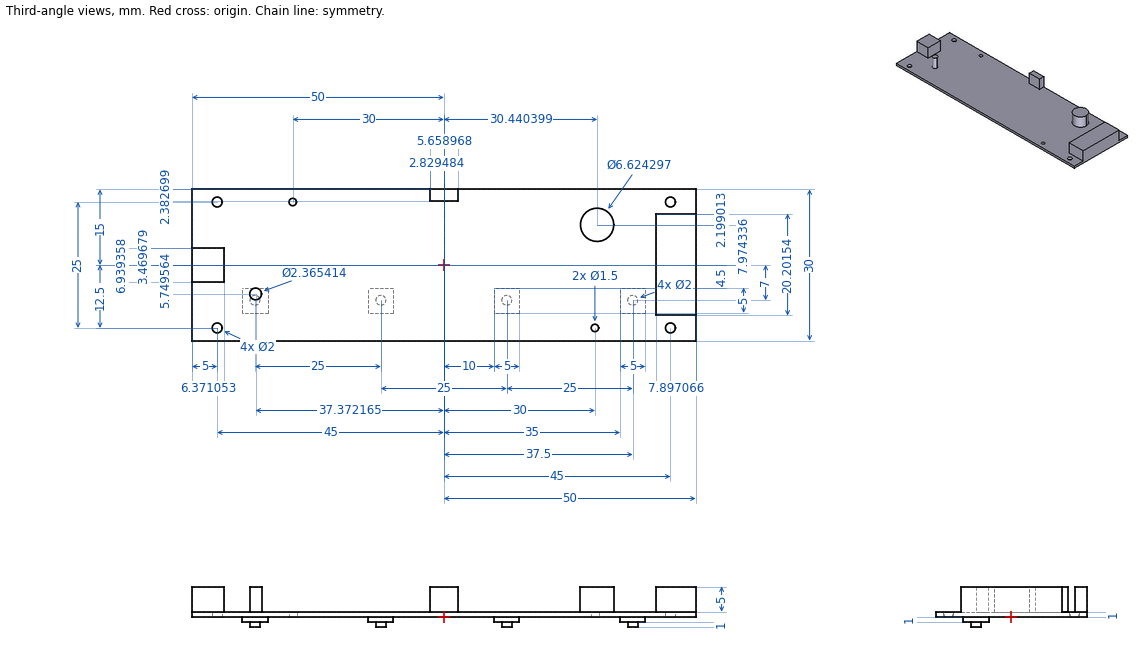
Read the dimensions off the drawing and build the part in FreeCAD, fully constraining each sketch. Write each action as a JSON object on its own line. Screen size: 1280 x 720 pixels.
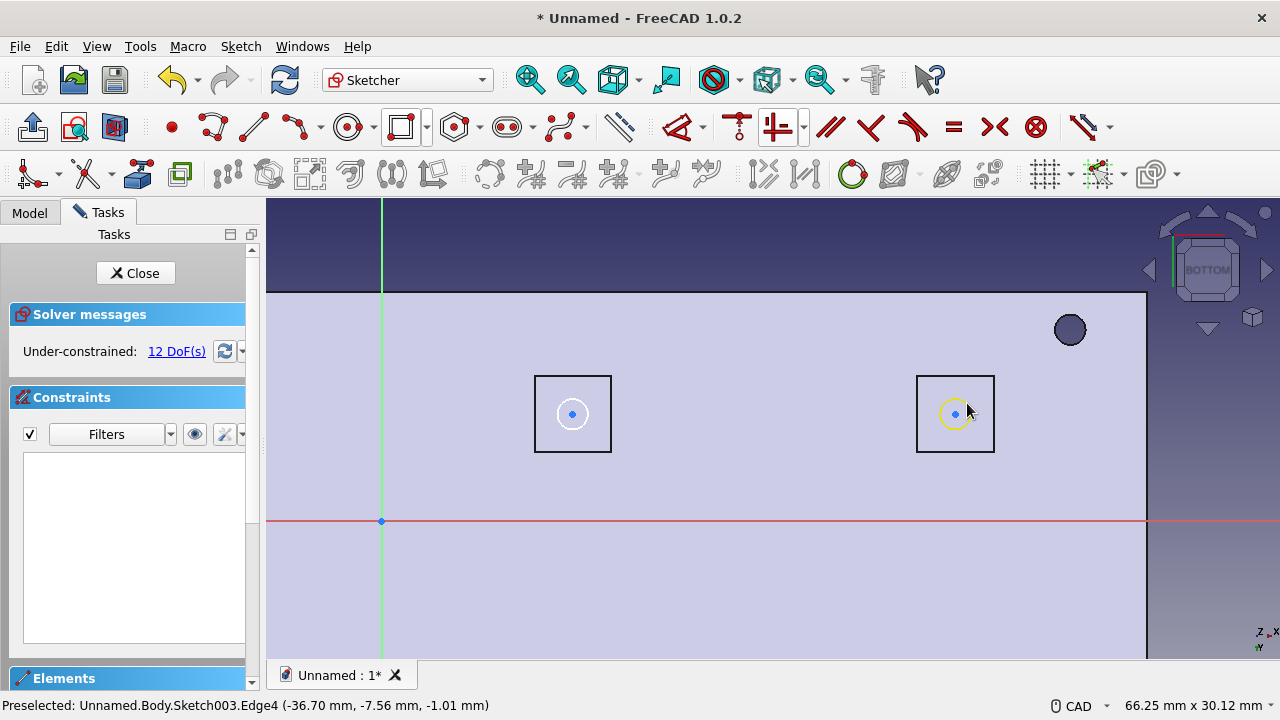
{"action": "left_click", "coordinate": [966, 404]}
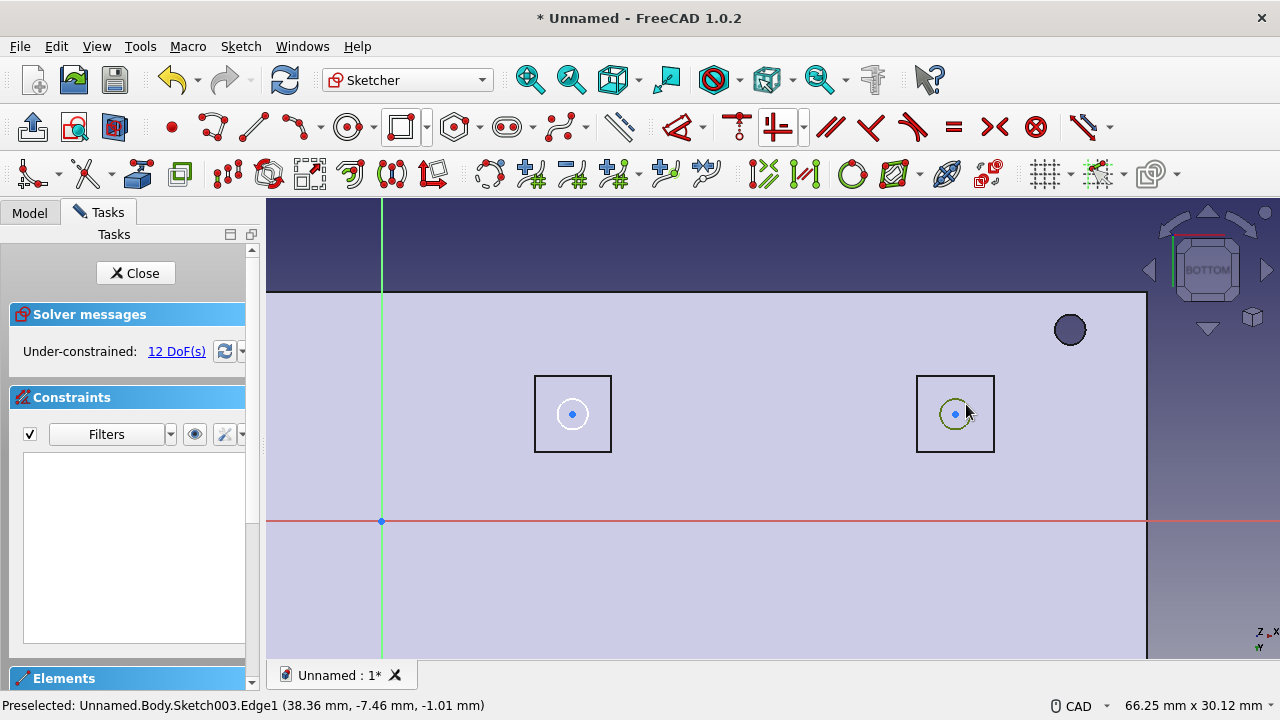
{"action": "left_click", "coordinate": [583, 404]}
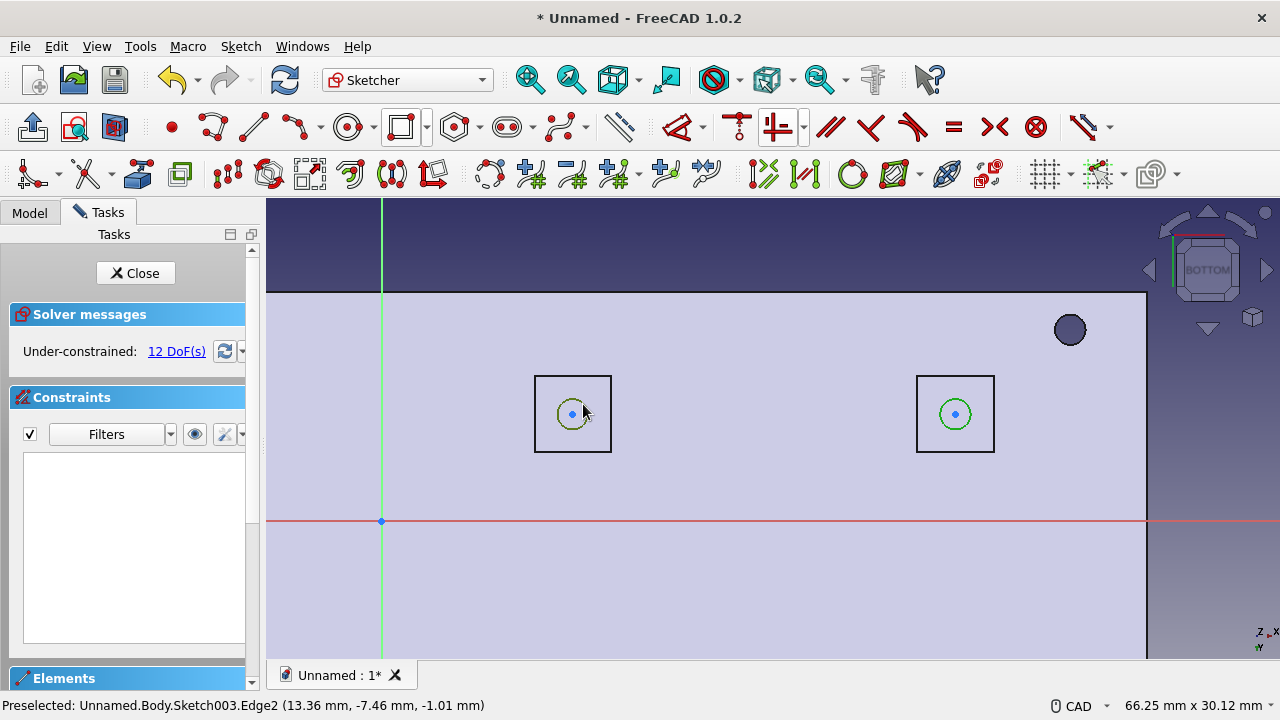
{"action": "scroll", "coordinate": [968, 403], "scroll_direction": "down", "scroll_amount": 4}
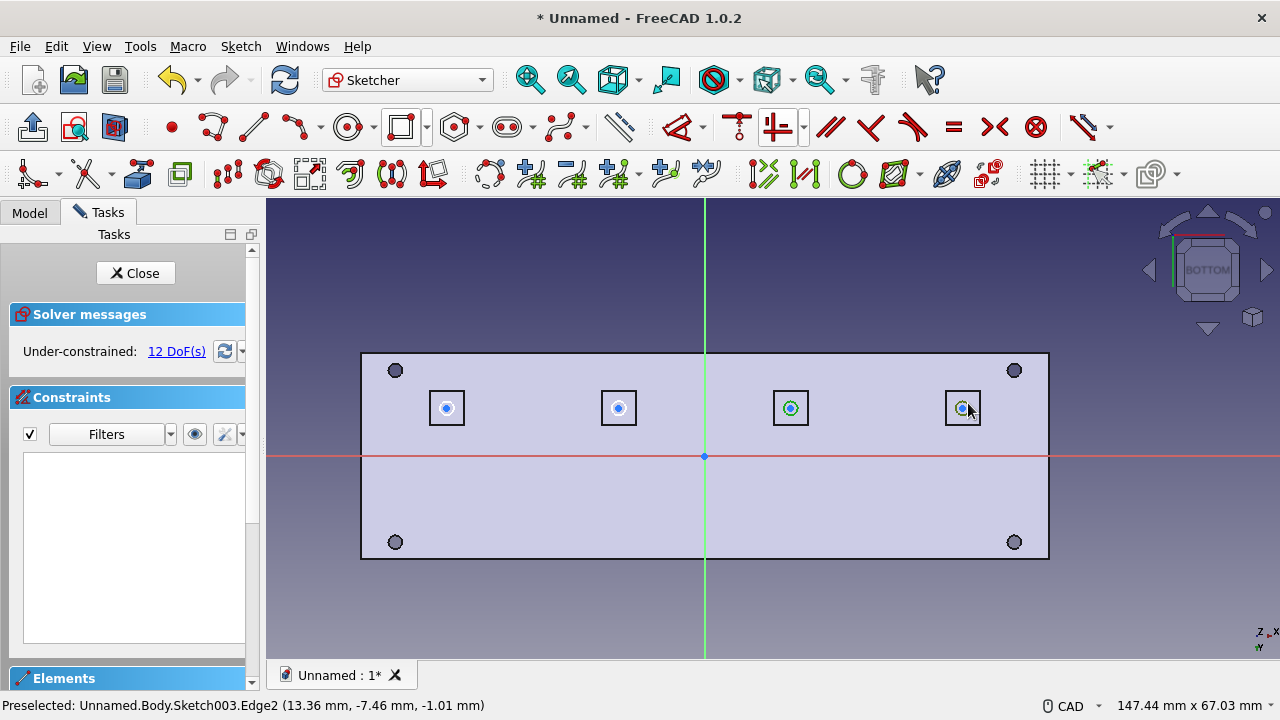
{"action": "scroll", "coordinate": [624, 403], "scroll_direction": "up", "scroll_amount": 4}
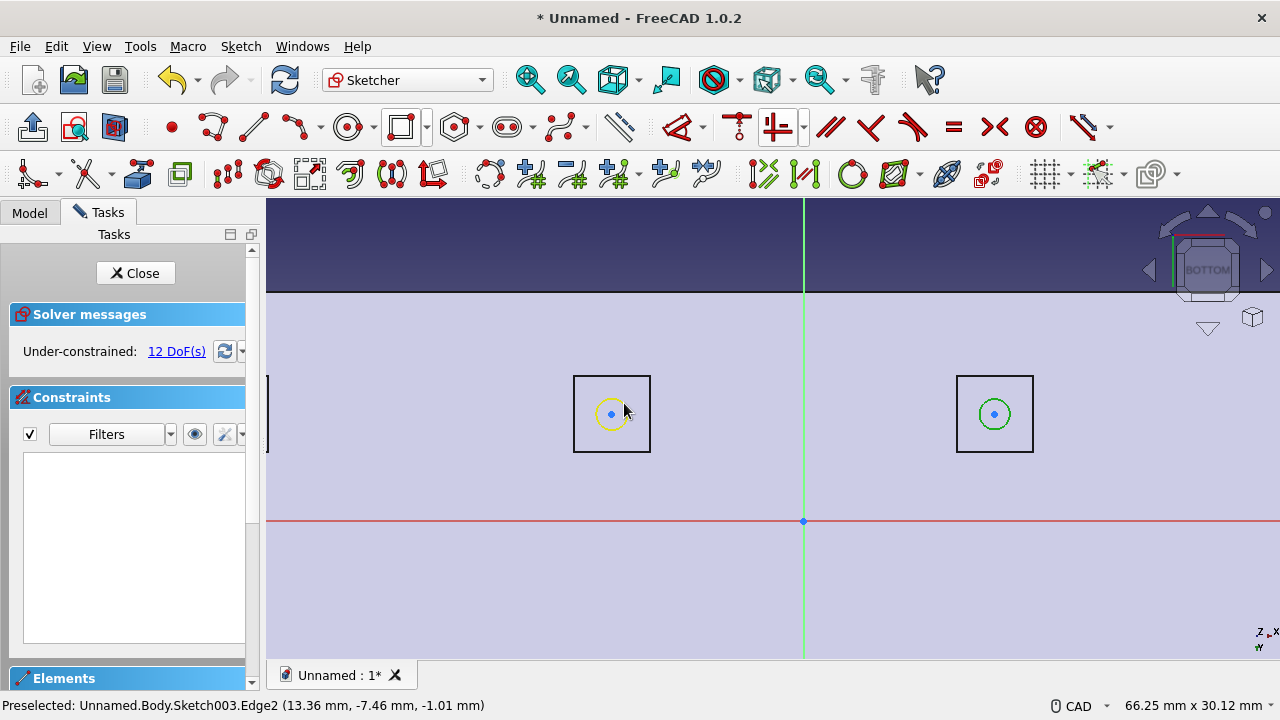
{"action": "left_click", "coordinate": [623, 403]}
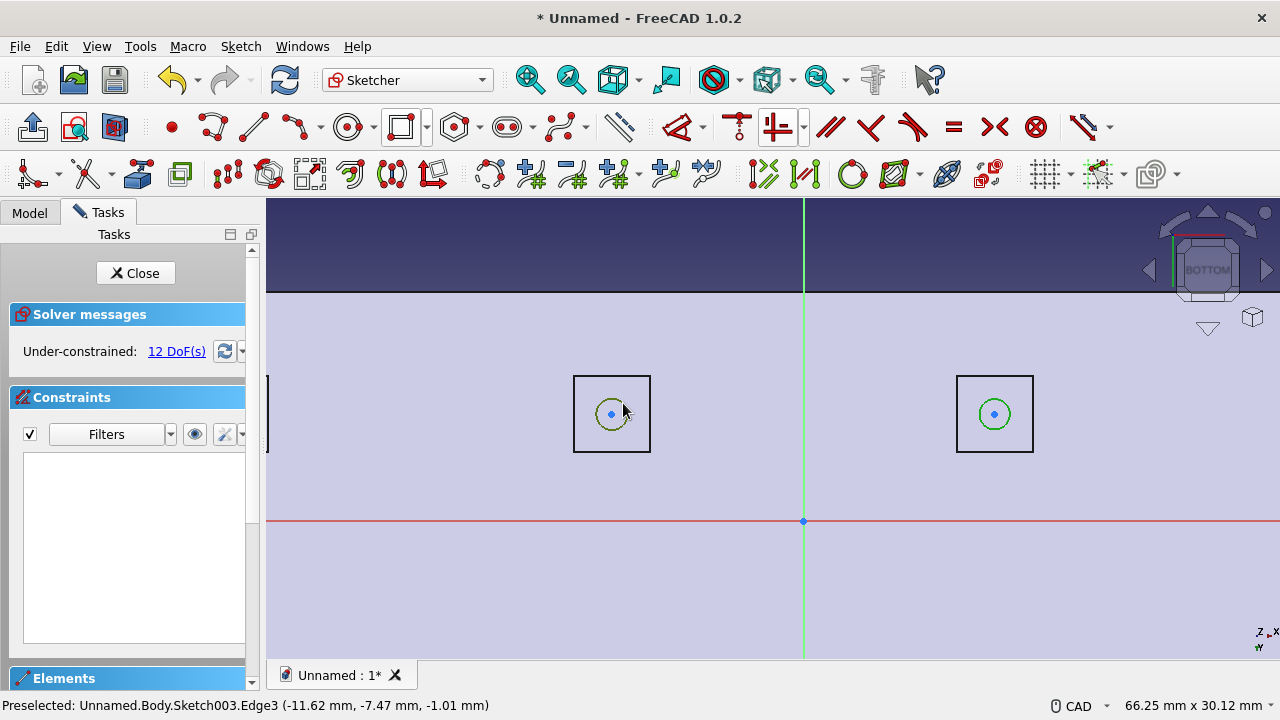
{"action": "scroll", "coordinate": [624, 403], "scroll_direction": "down", "scroll_amount": 4}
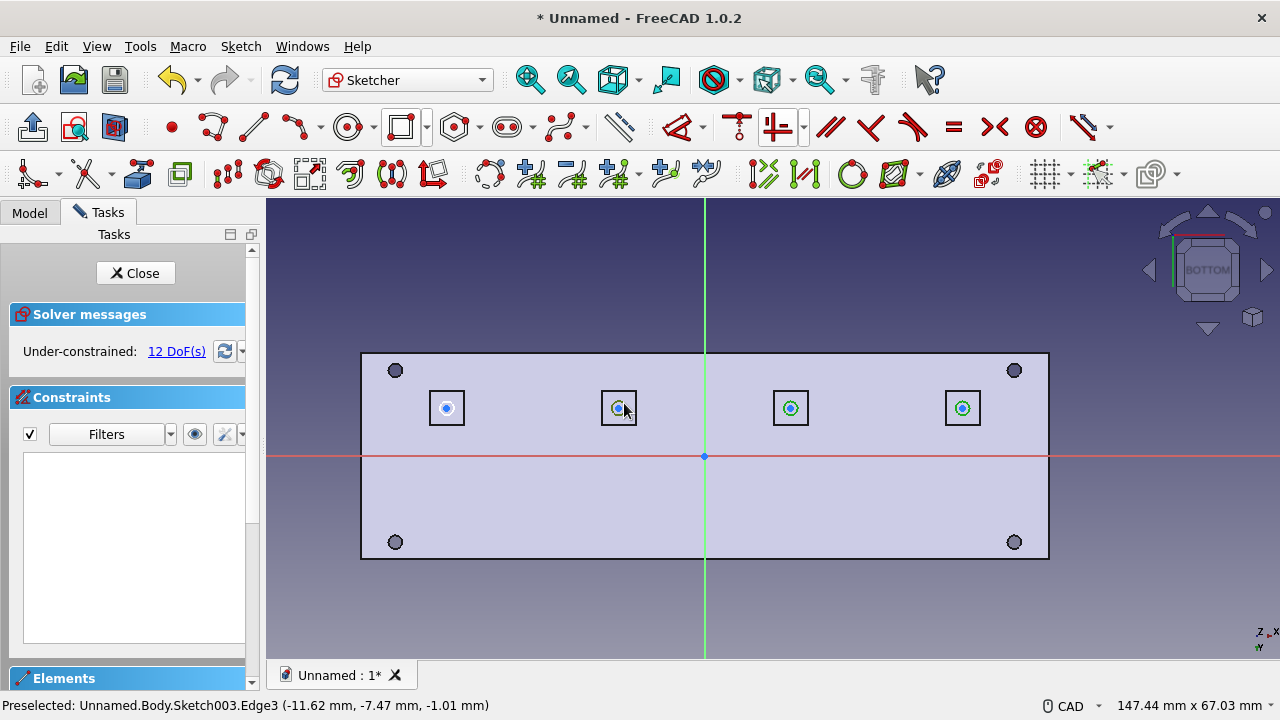
{"action": "scroll", "coordinate": [452, 403], "scroll_direction": "up", "scroll_amount": 4}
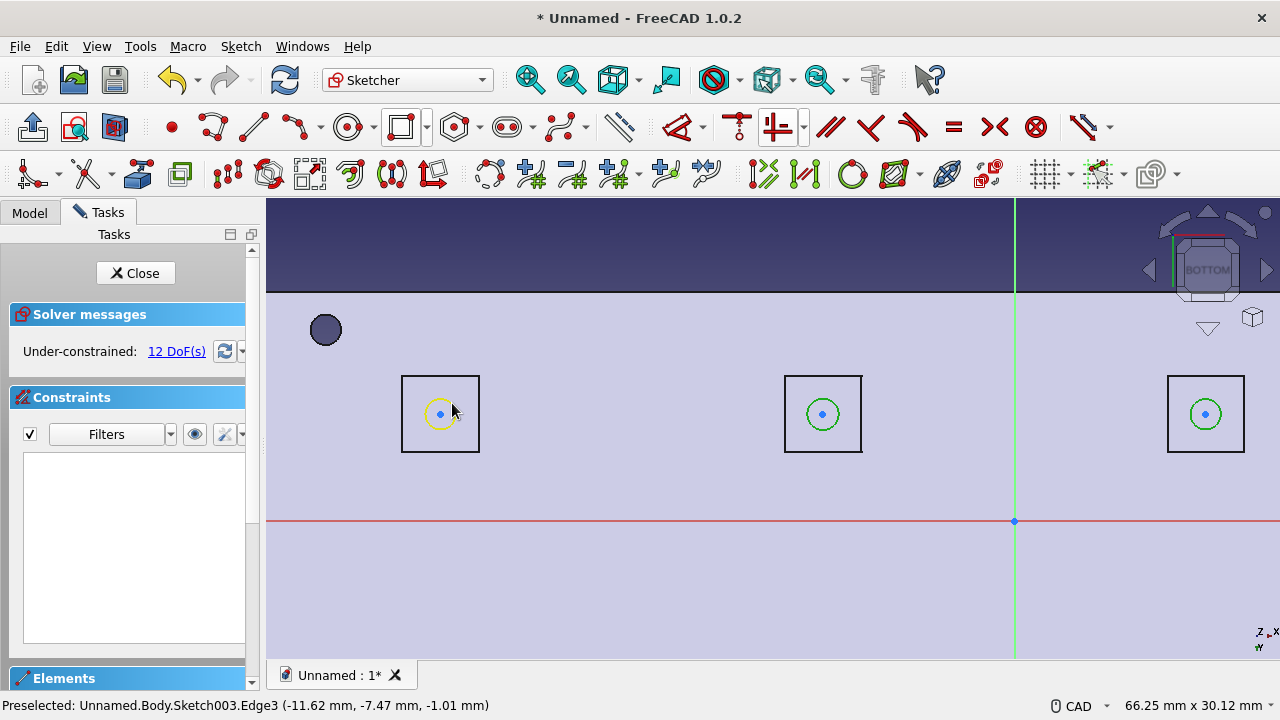
{"action": "left_click", "coordinate": [451, 404]}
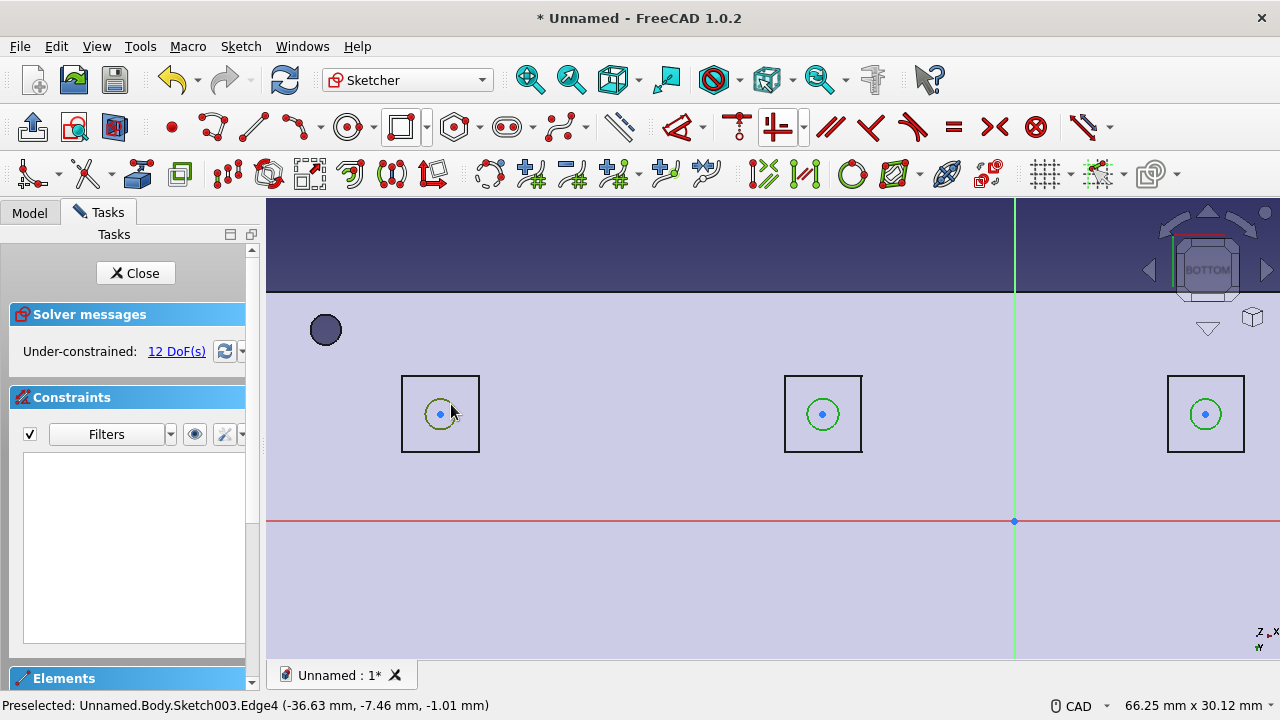
{"action": "left_click", "coordinate": [954, 128]}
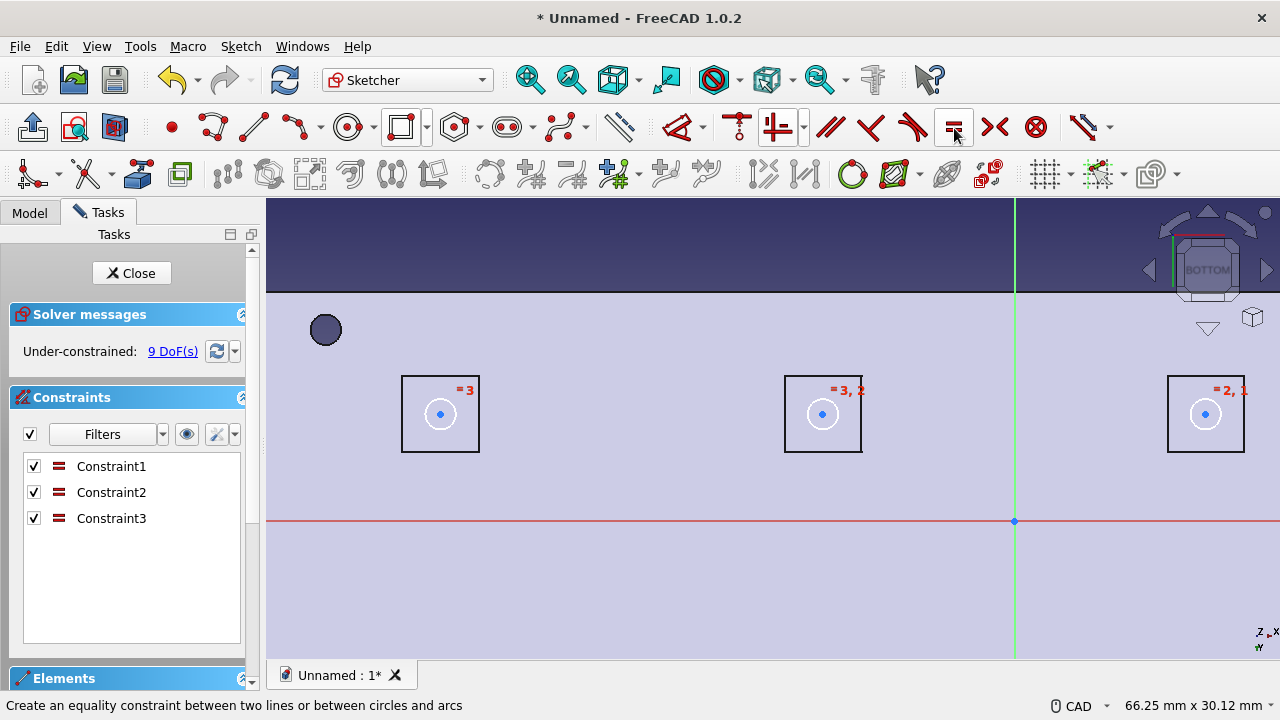
{"action": "scroll", "coordinate": [452, 403], "scroll_direction": "down", "scroll_amount": 4}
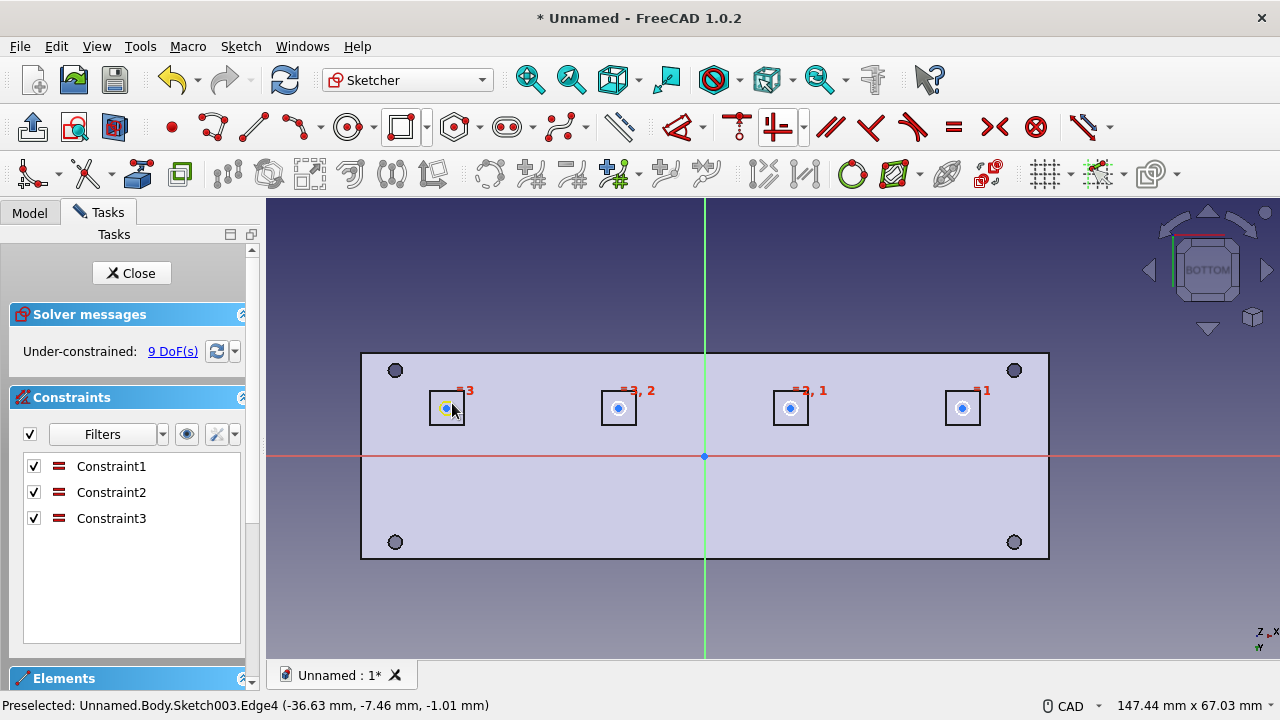
{"action": "left_click", "coordinate": [963, 408]}